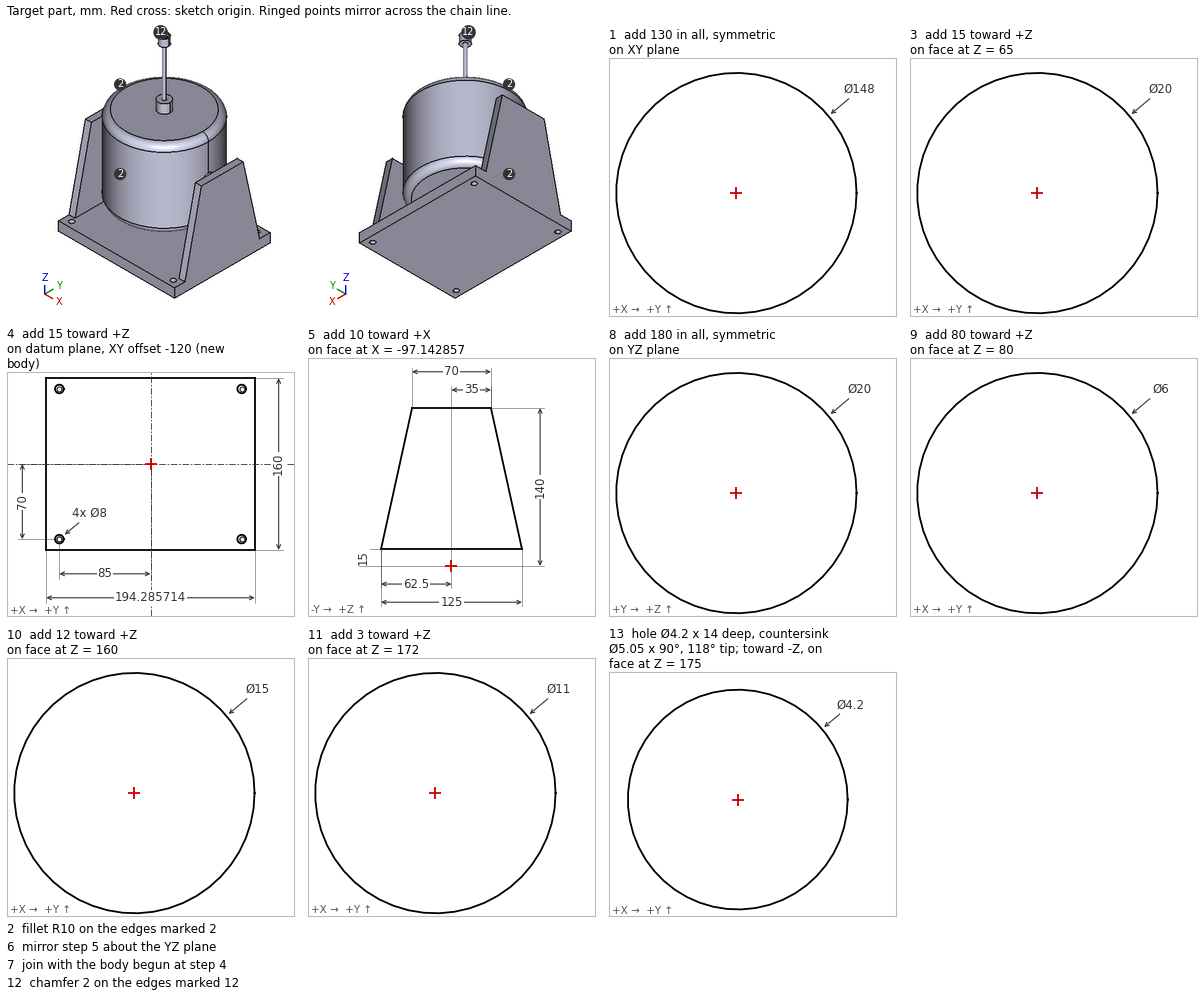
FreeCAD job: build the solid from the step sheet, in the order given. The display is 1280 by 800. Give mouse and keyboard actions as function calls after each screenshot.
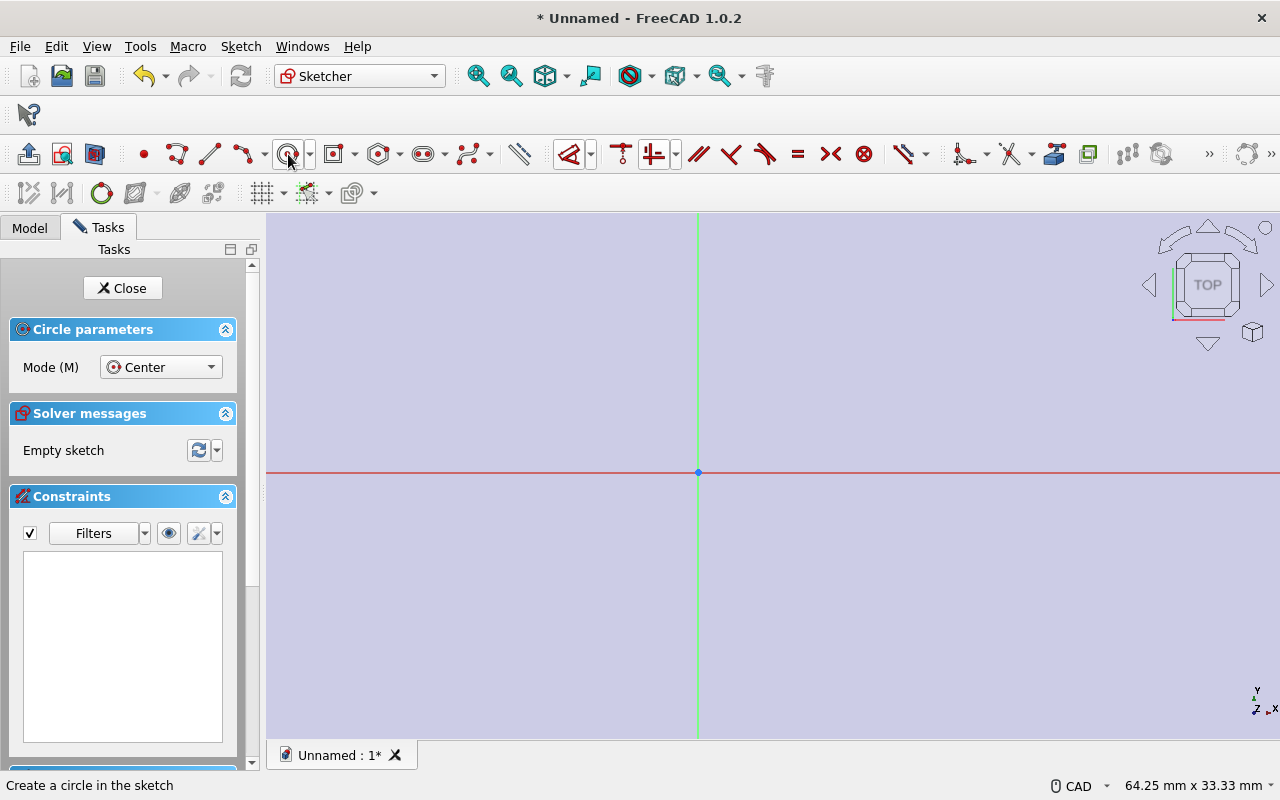
click(698, 473)
click(810, 361)
key(Escape)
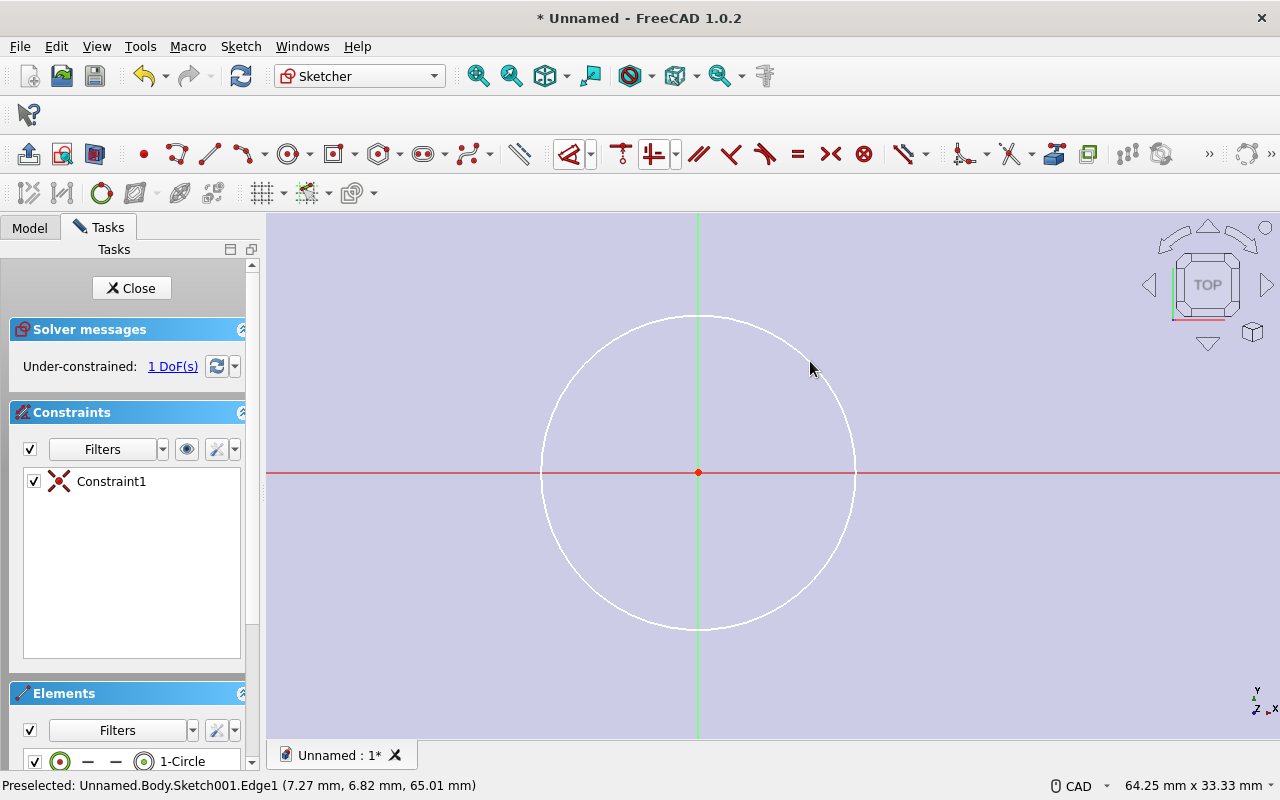
click(809, 361)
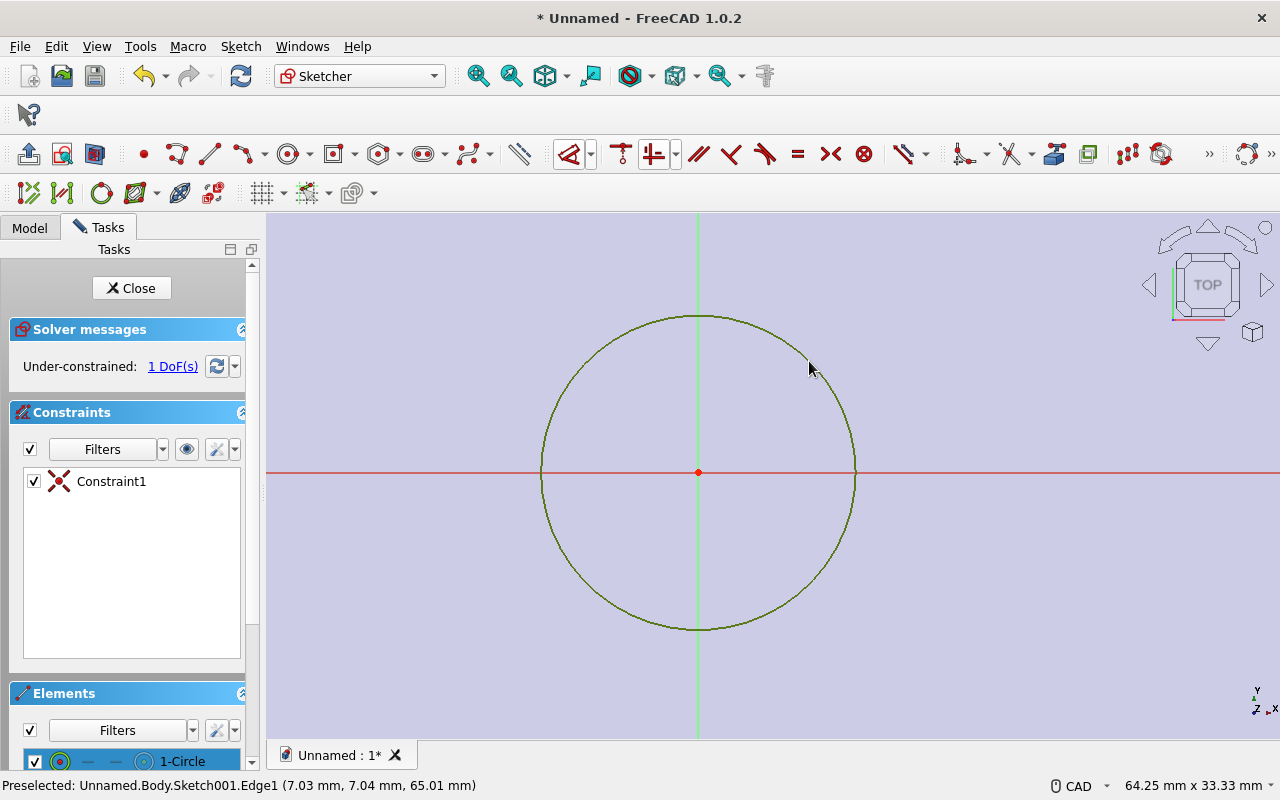
key(k)
key(o)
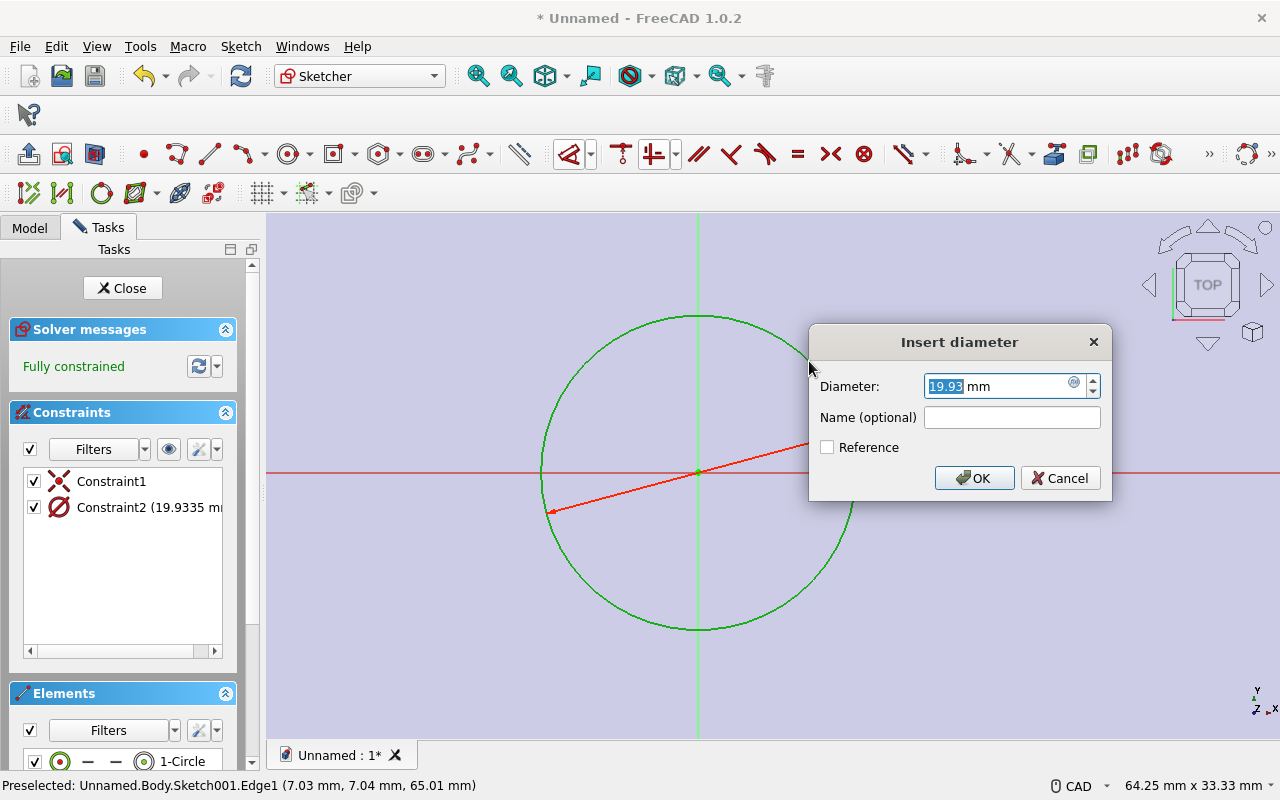
text(20)
key(Return)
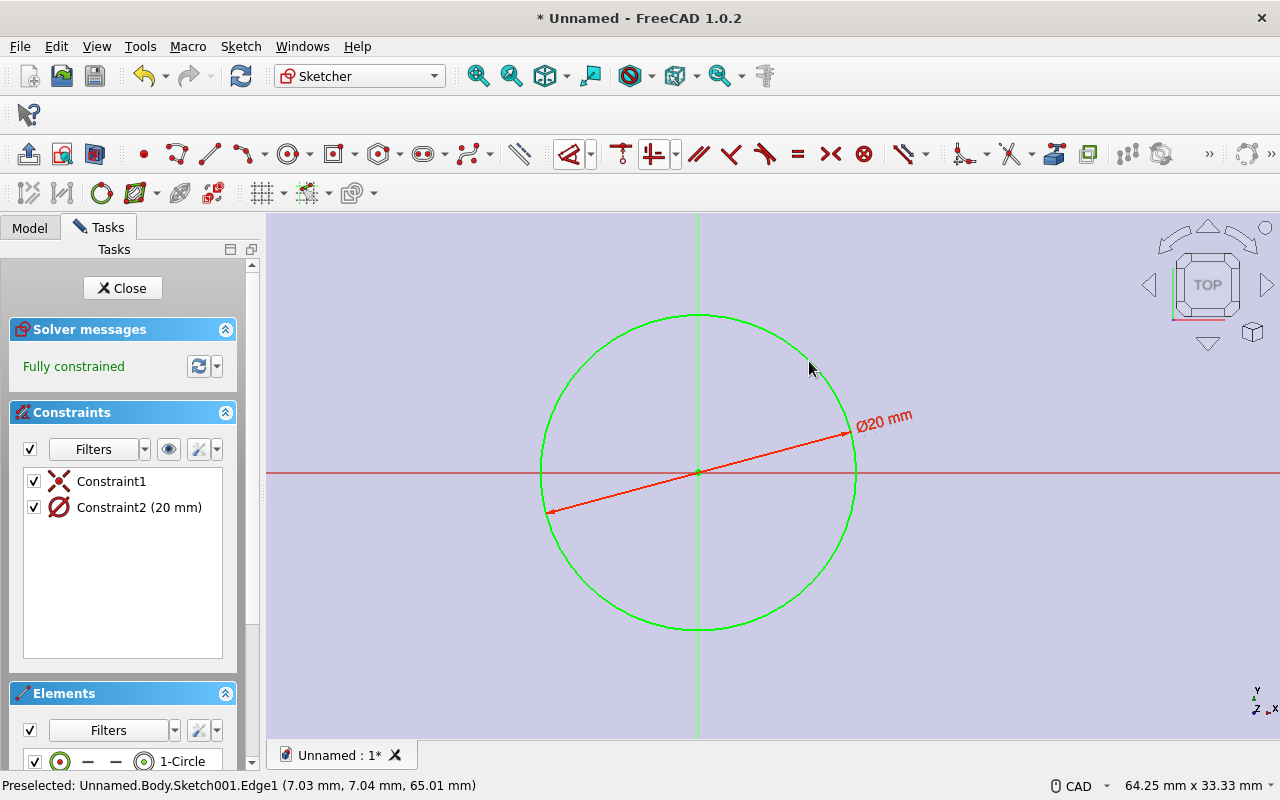
click(123, 288)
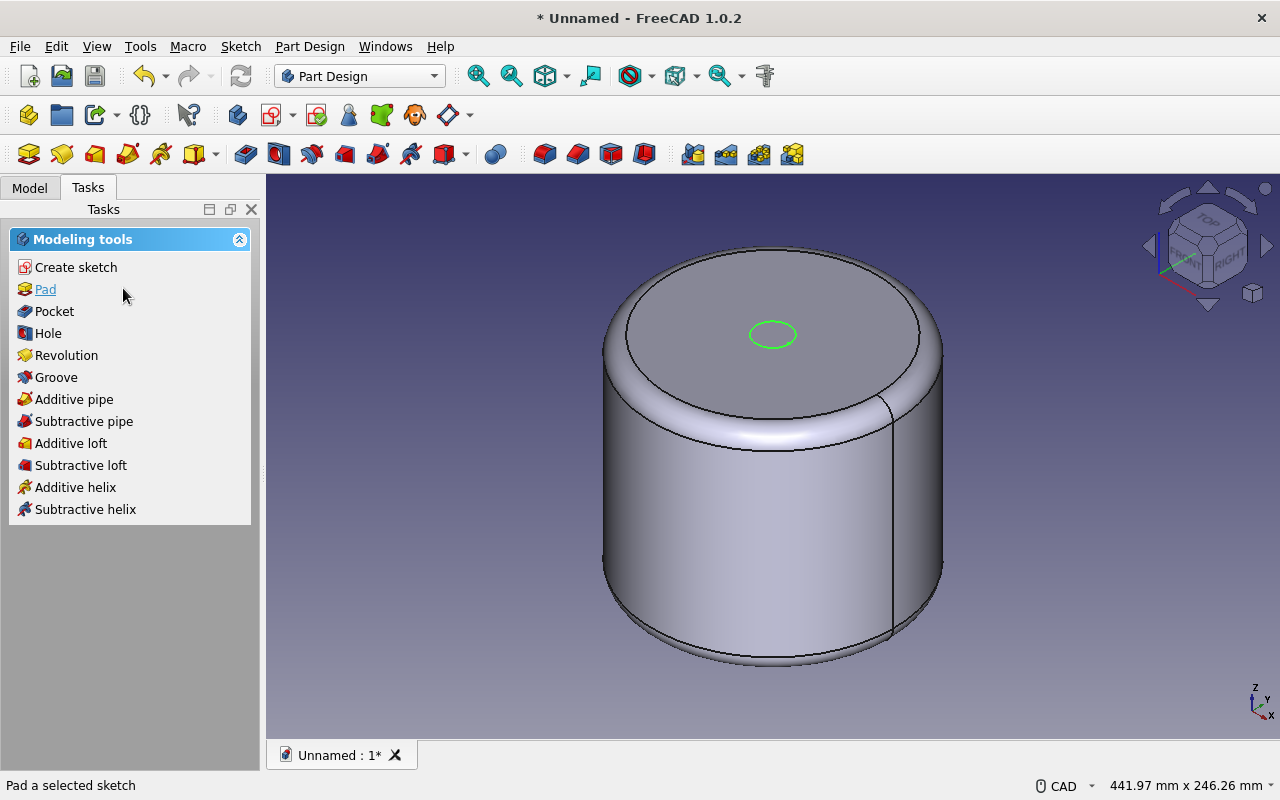
click(29, 154)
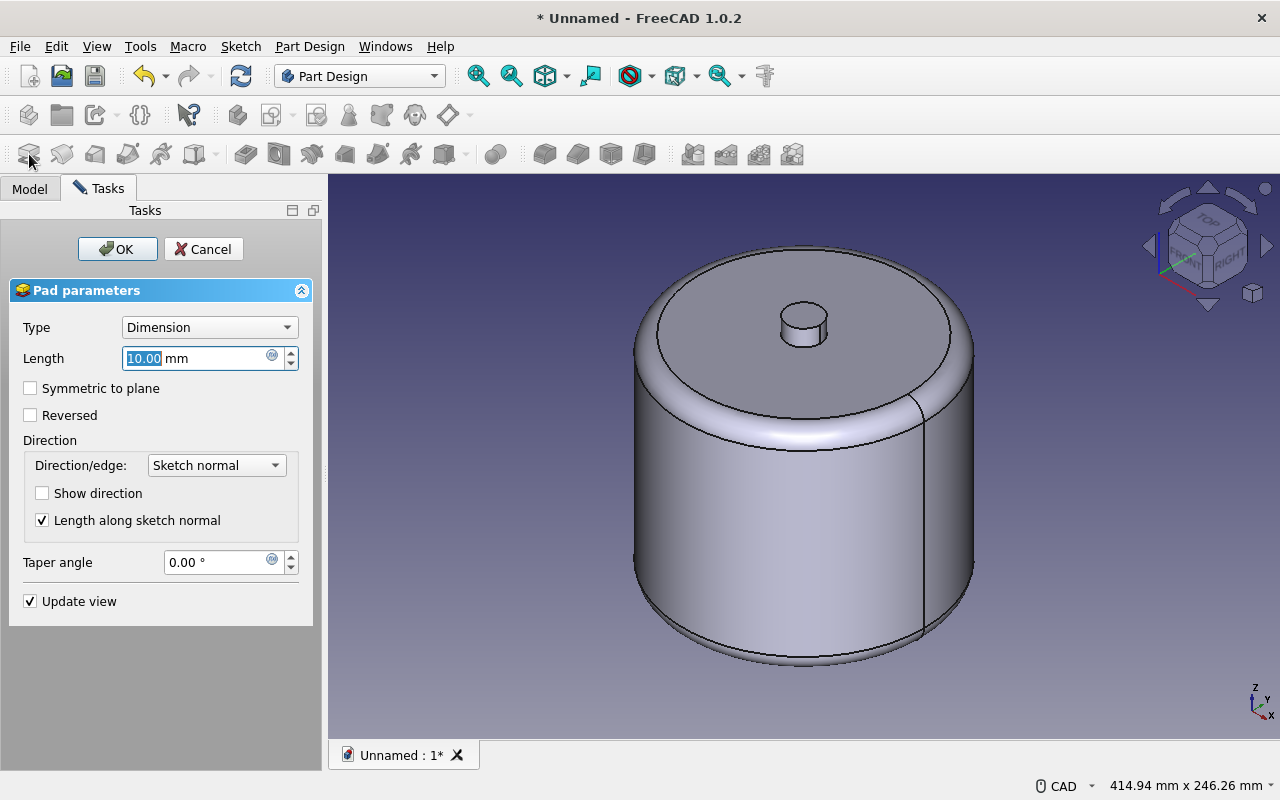
text(15)
key(Tab)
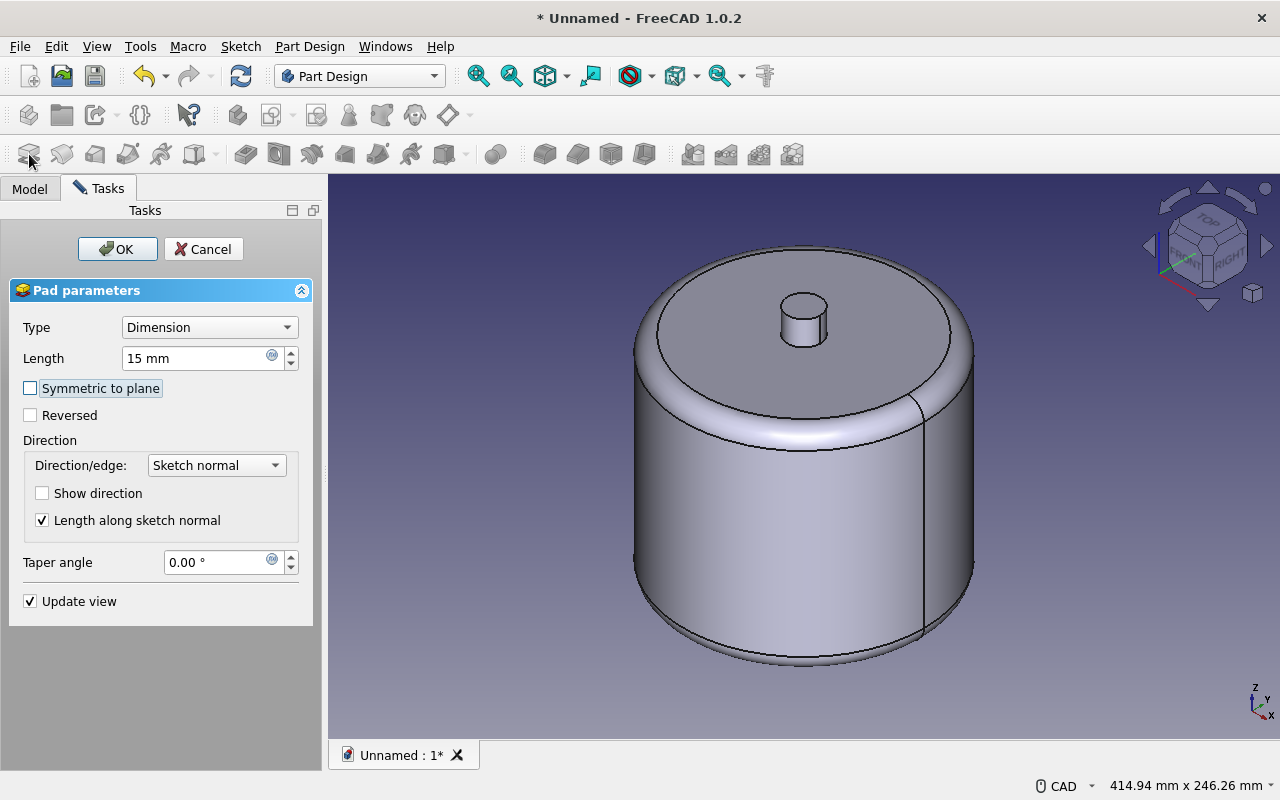
click(118, 249)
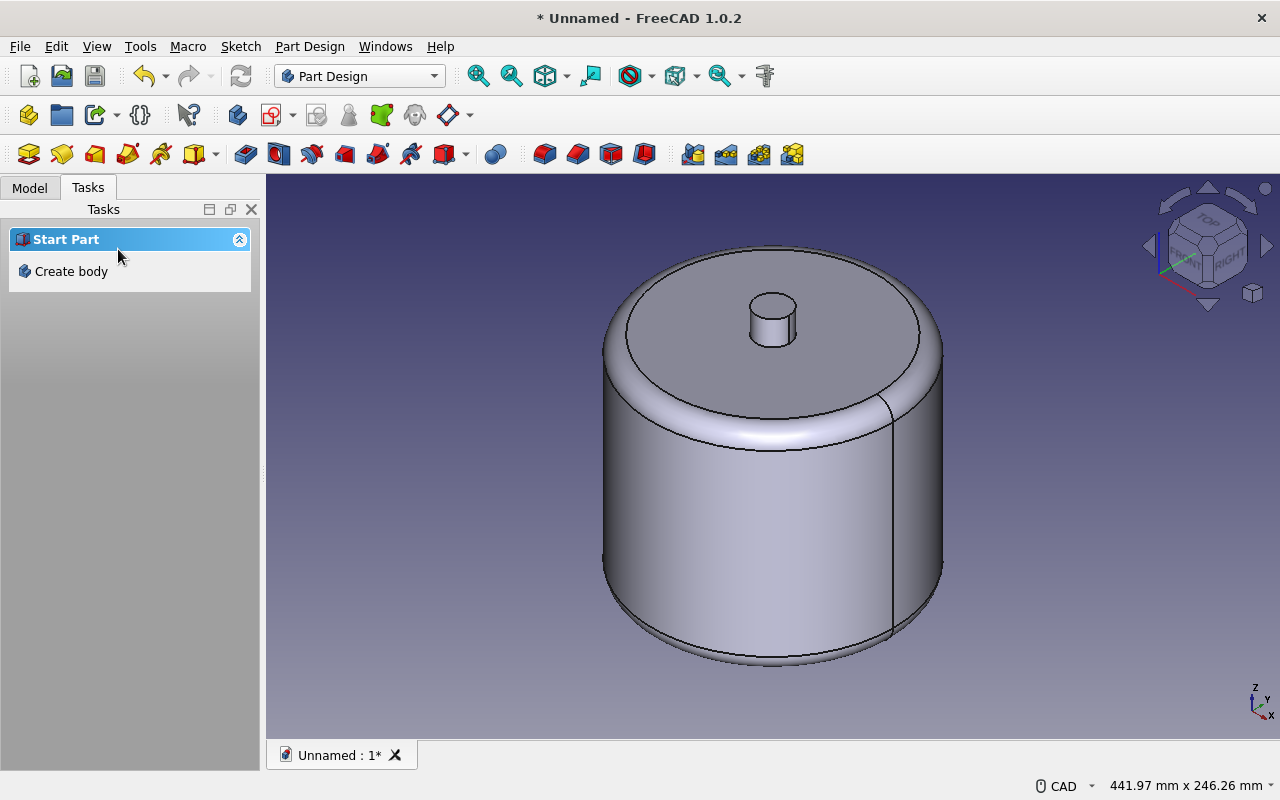
key(v)
key(f)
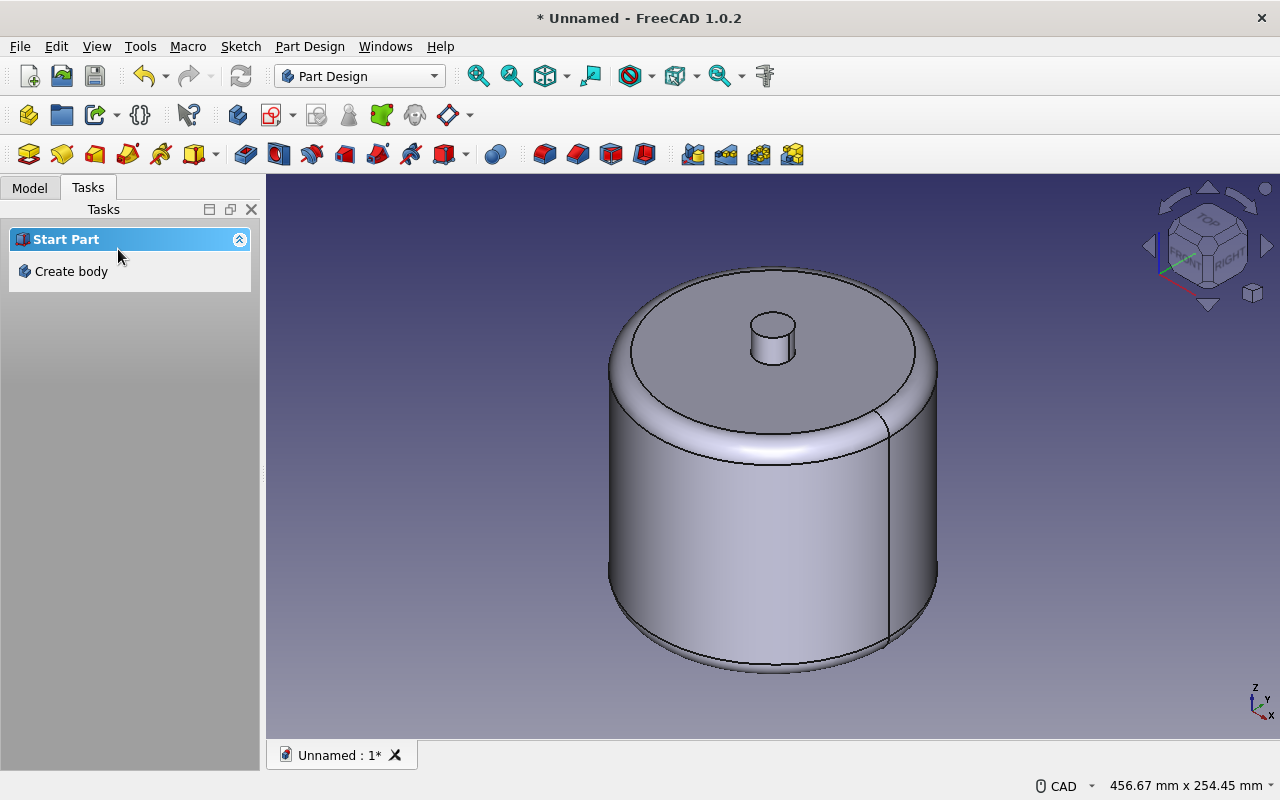
click(238, 116)